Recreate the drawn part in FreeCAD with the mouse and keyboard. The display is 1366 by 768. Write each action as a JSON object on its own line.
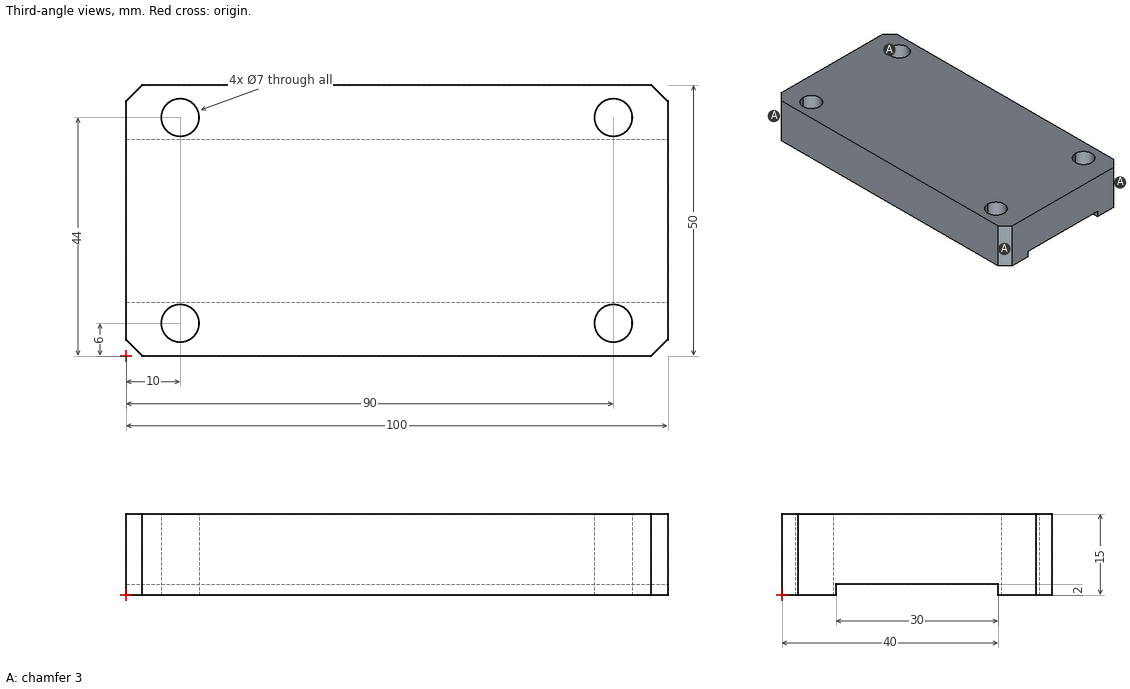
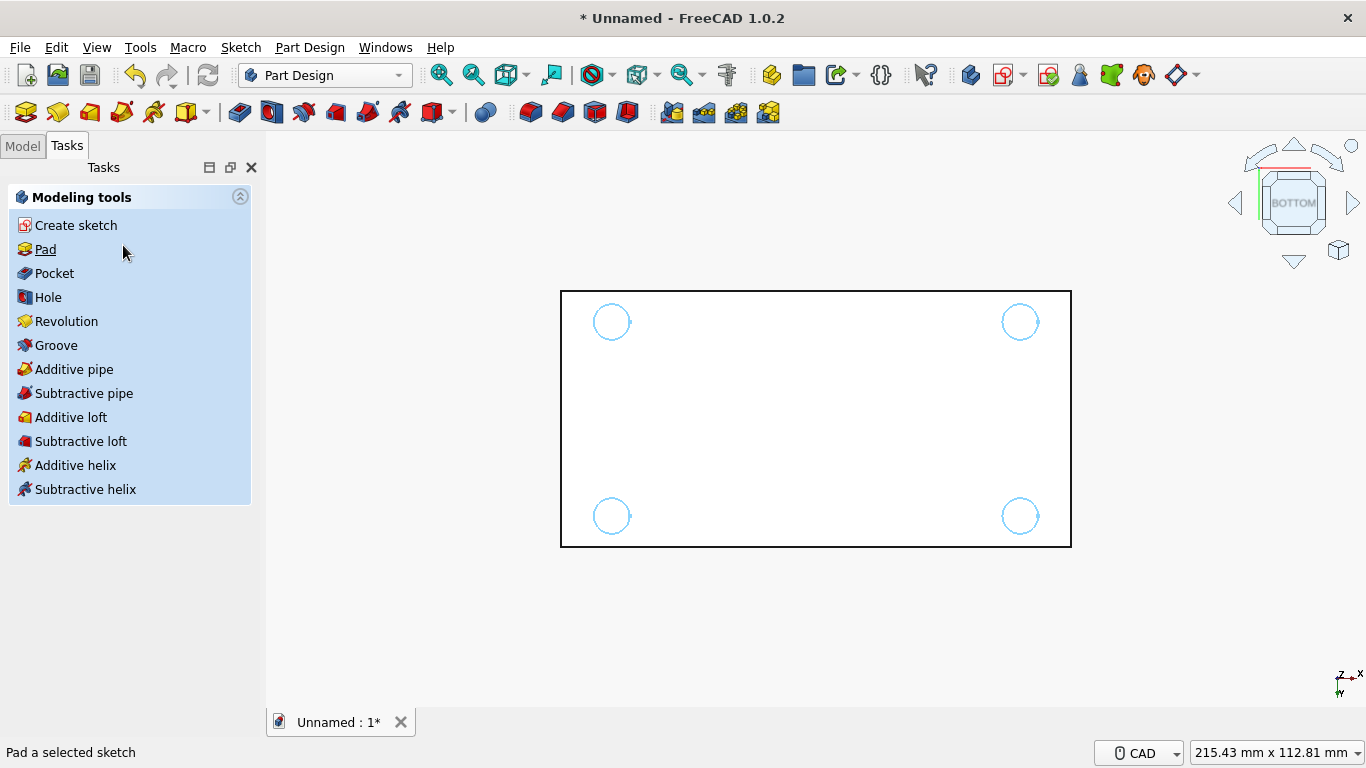
{"action": "left_click", "coordinate": [272, 112]}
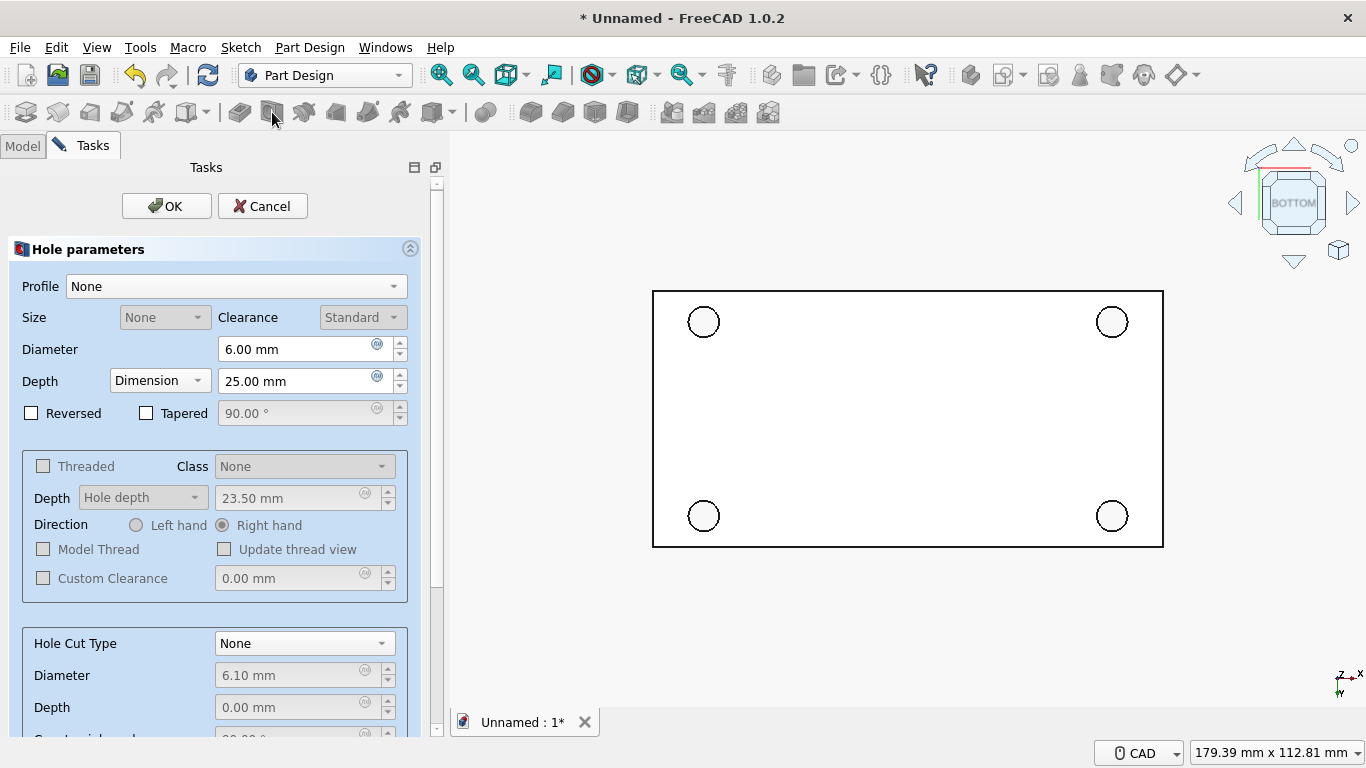
{"action": "triple_click", "coordinate": [305, 349]}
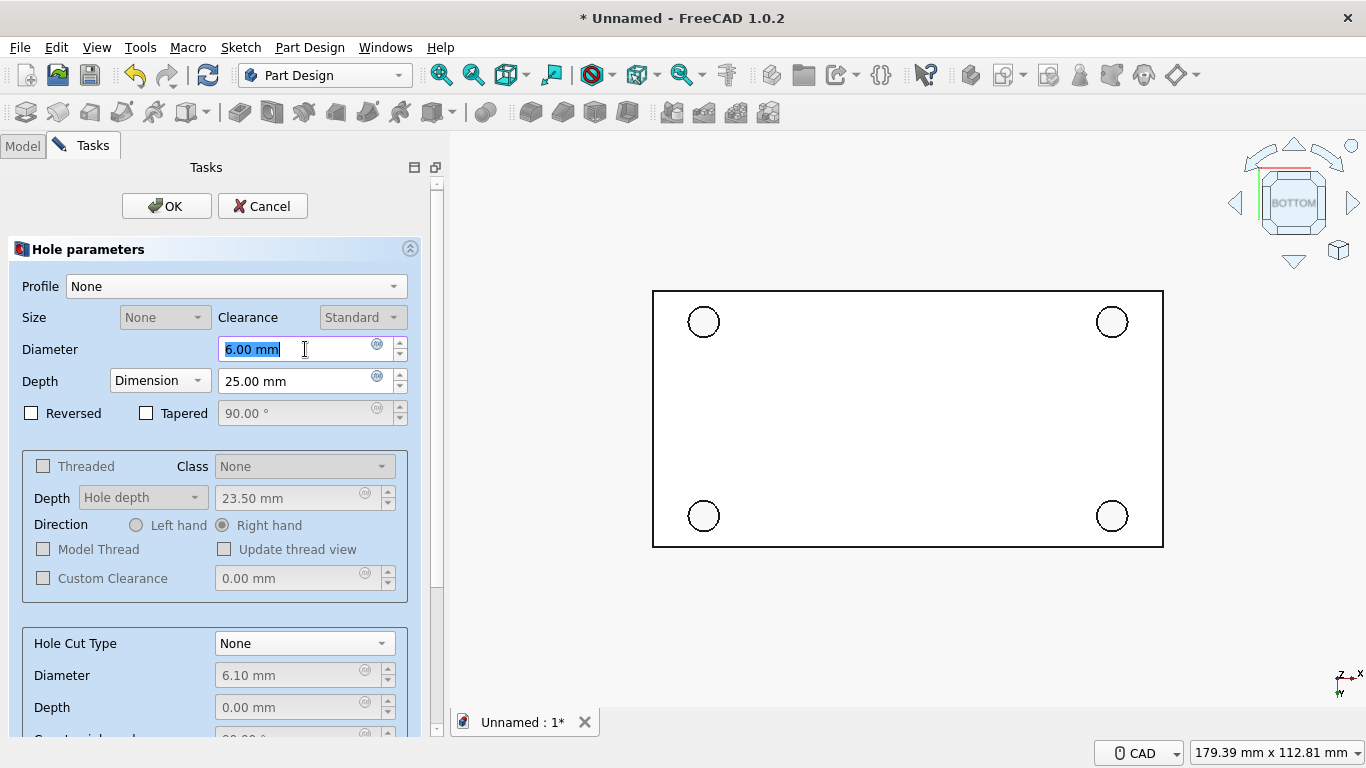
{"action": "type", "text": "7"}
{"action": "key", "text": "Tab"}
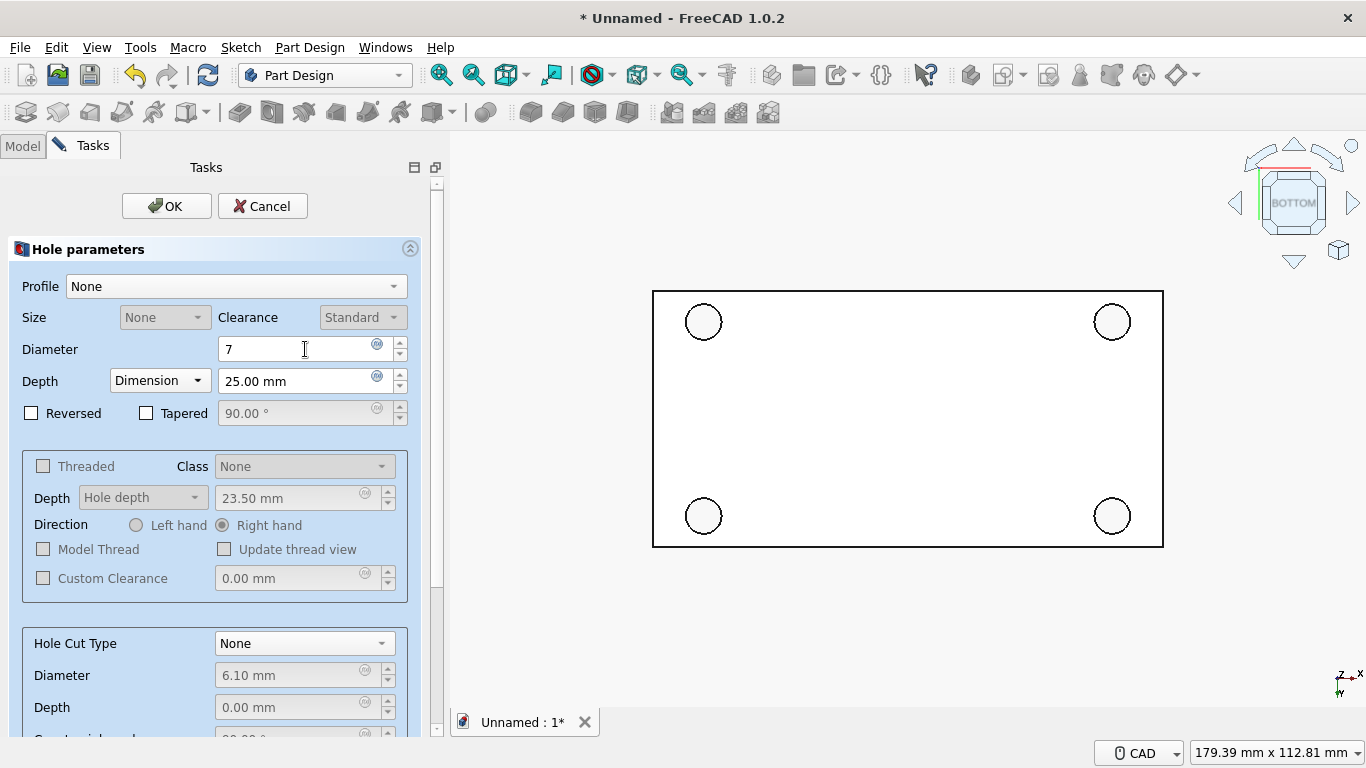
{"action": "left_click", "coordinate": [161, 380]}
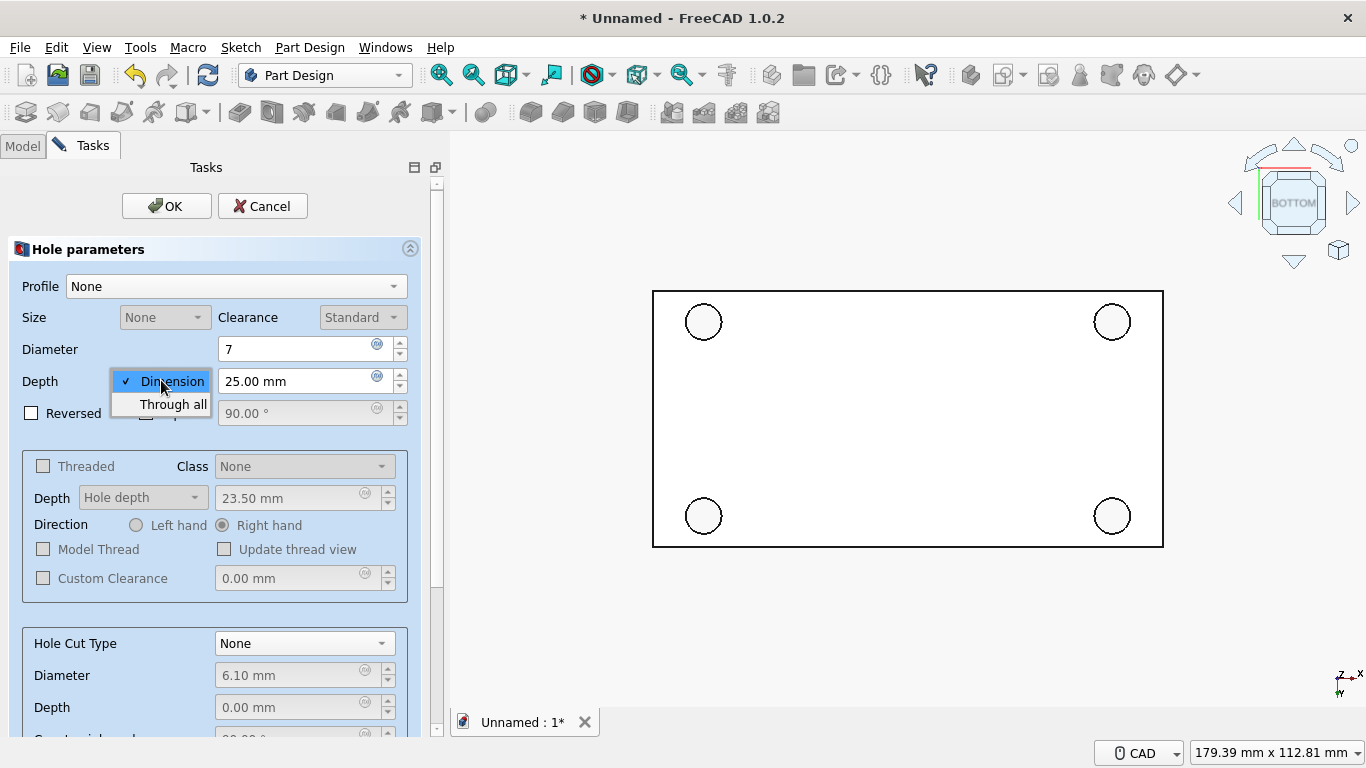
{"action": "left_click", "coordinate": [160, 404]}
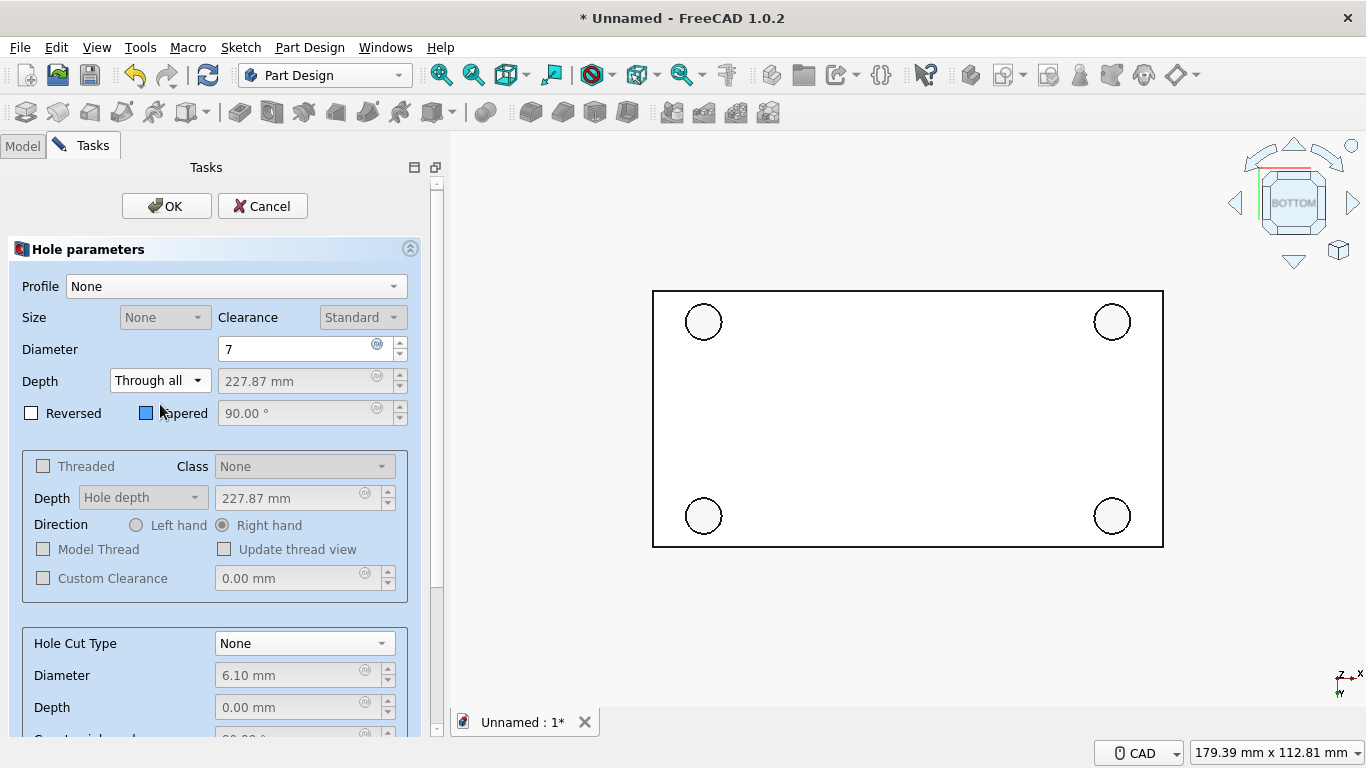
{"action": "left_click", "coordinate": [167, 206]}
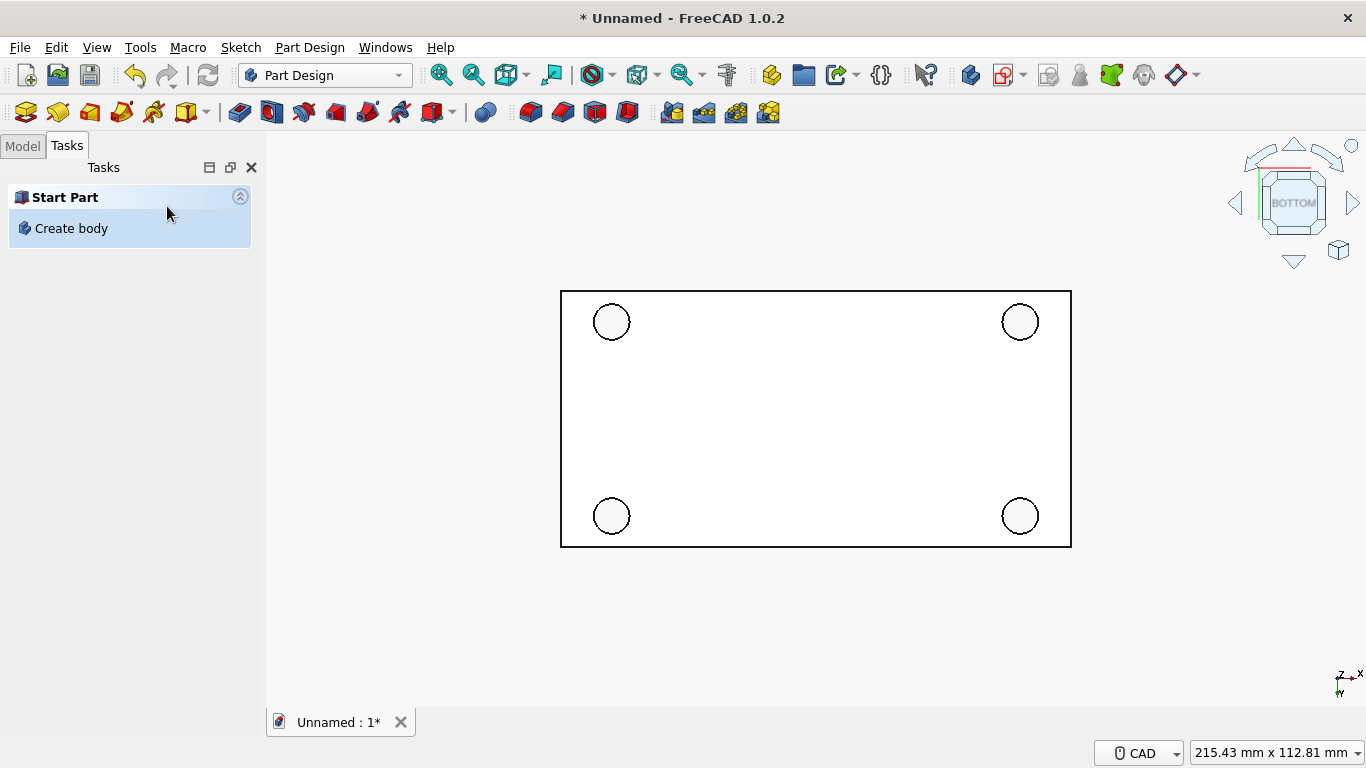
{"action": "key", "text": "0"}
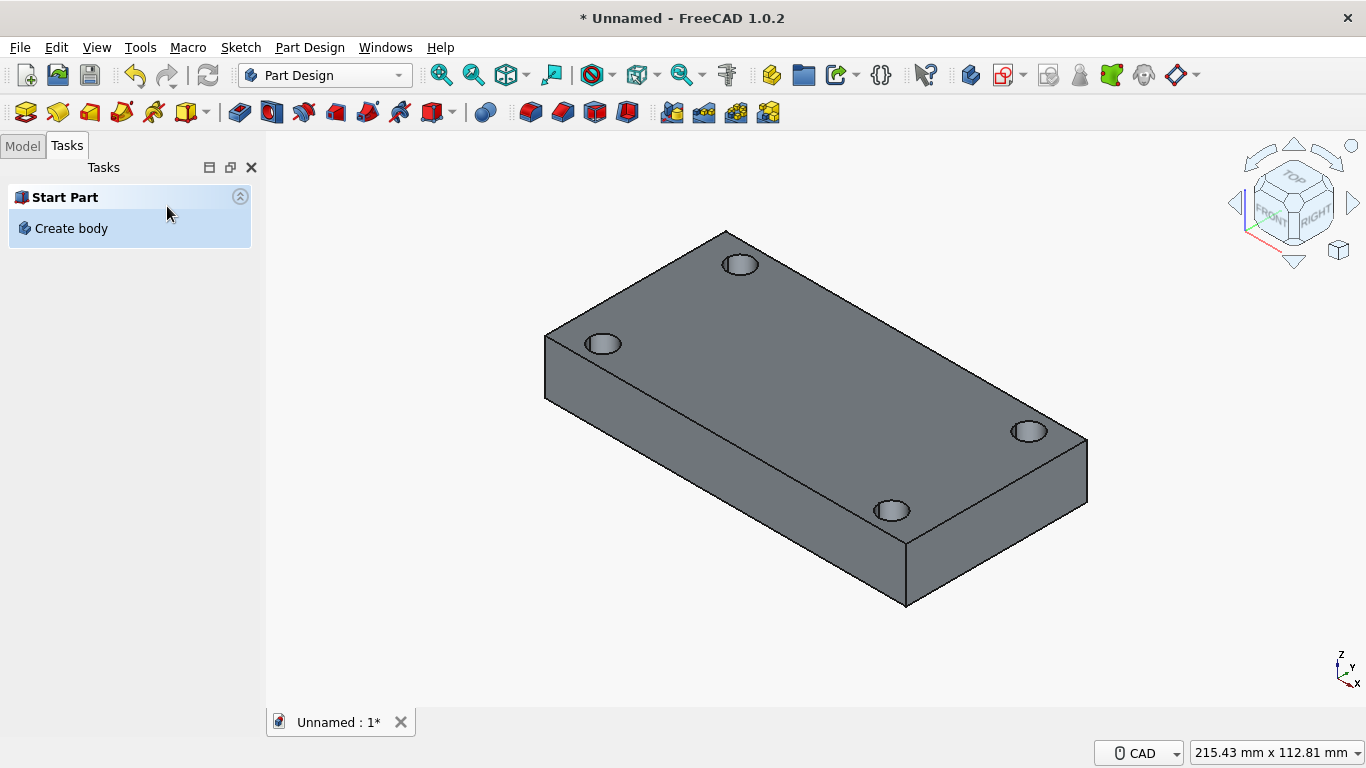
{"action": "left_click", "coordinate": [906, 574]}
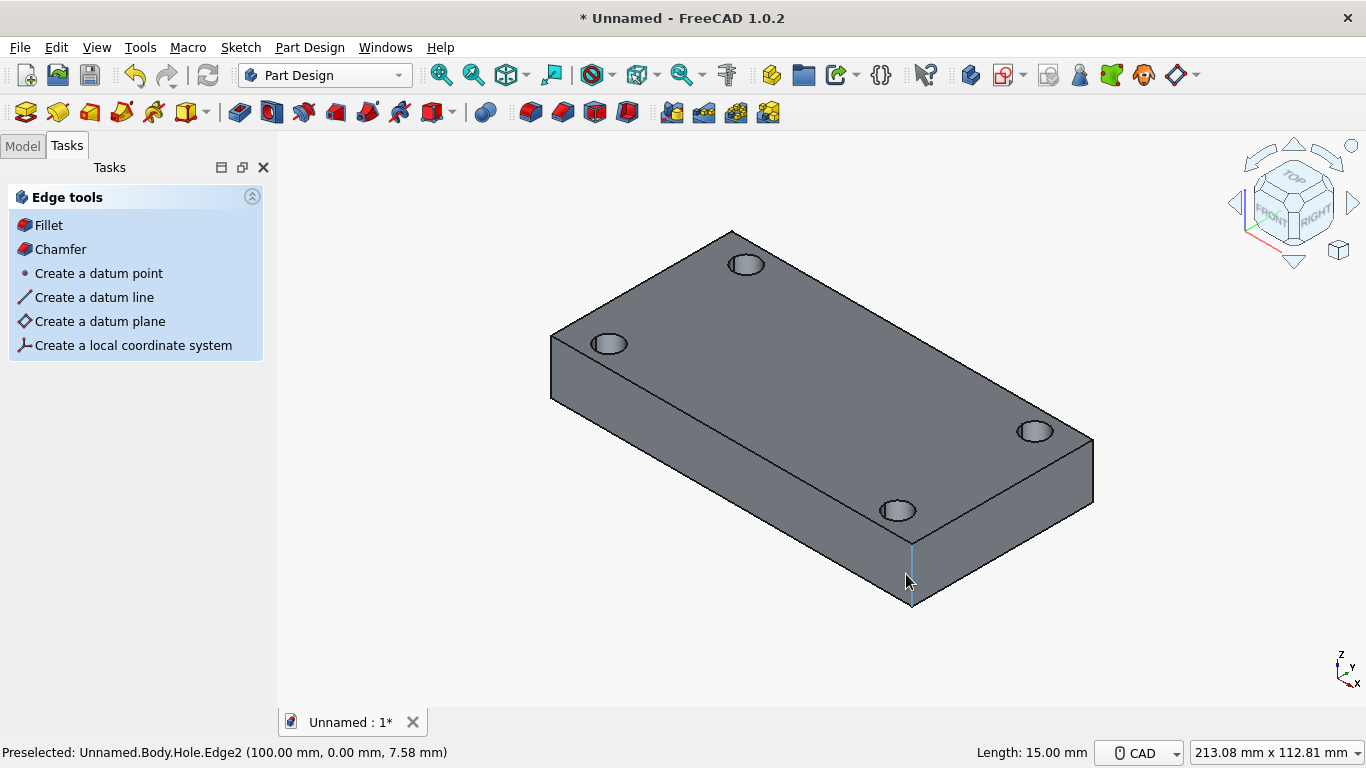
{"action": "key", "text": "2"}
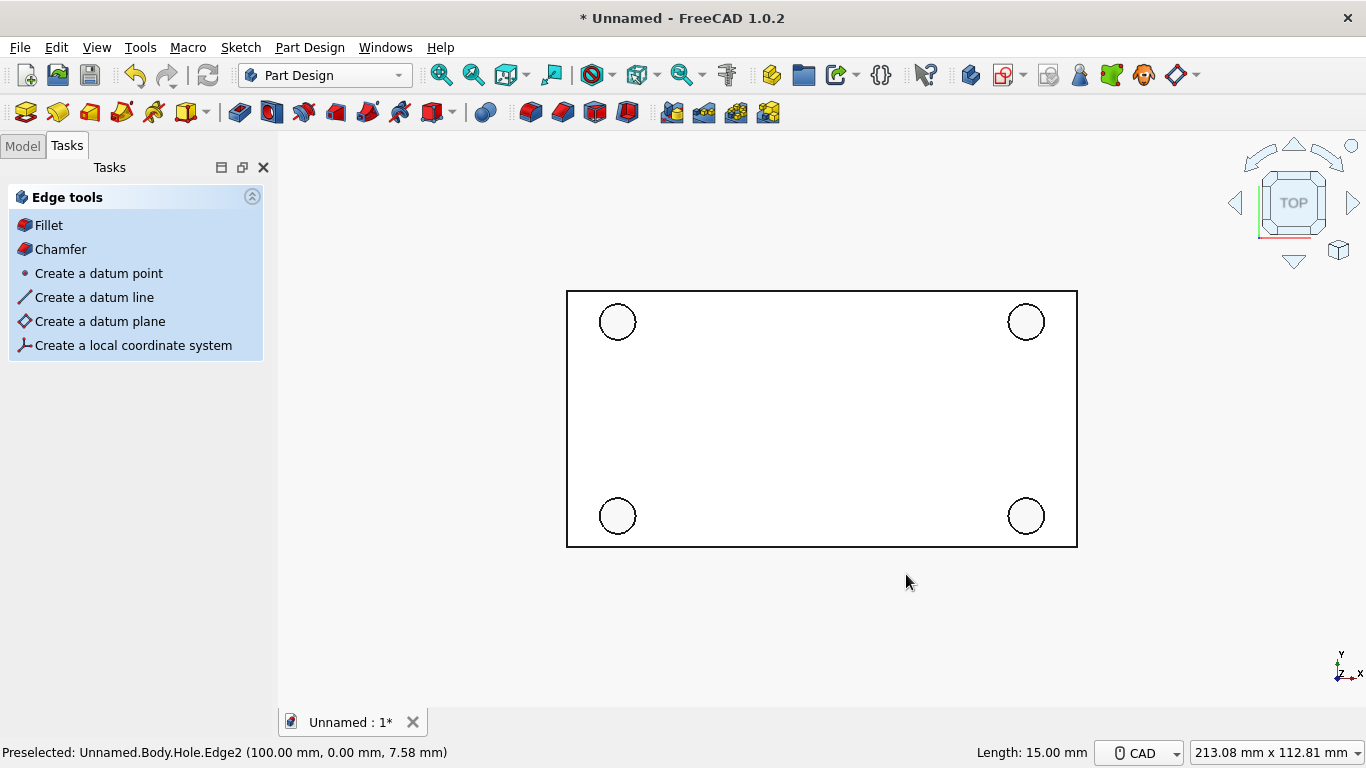
{"action": "key", "text": "1"}